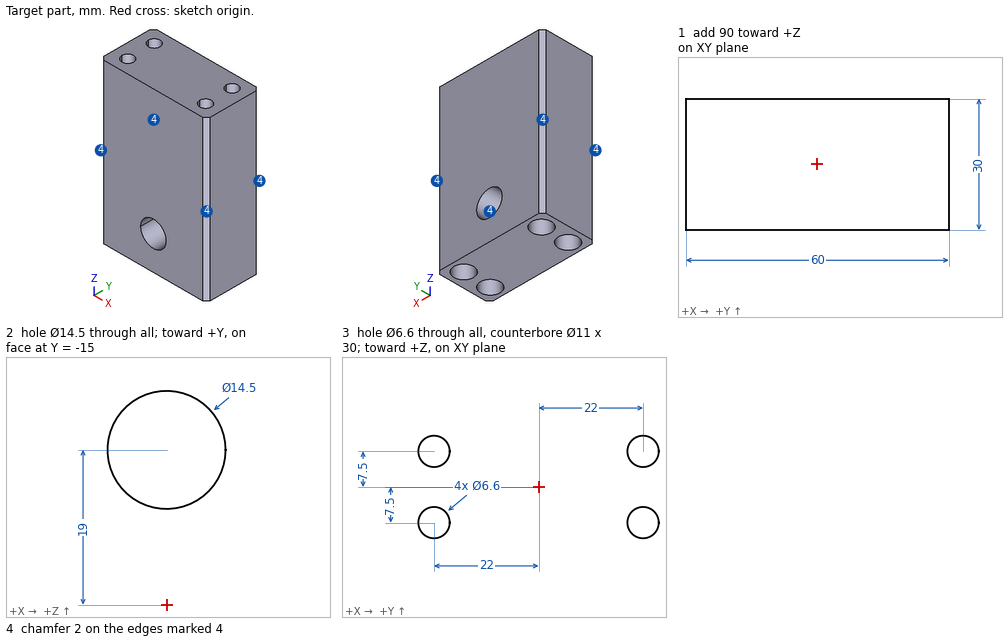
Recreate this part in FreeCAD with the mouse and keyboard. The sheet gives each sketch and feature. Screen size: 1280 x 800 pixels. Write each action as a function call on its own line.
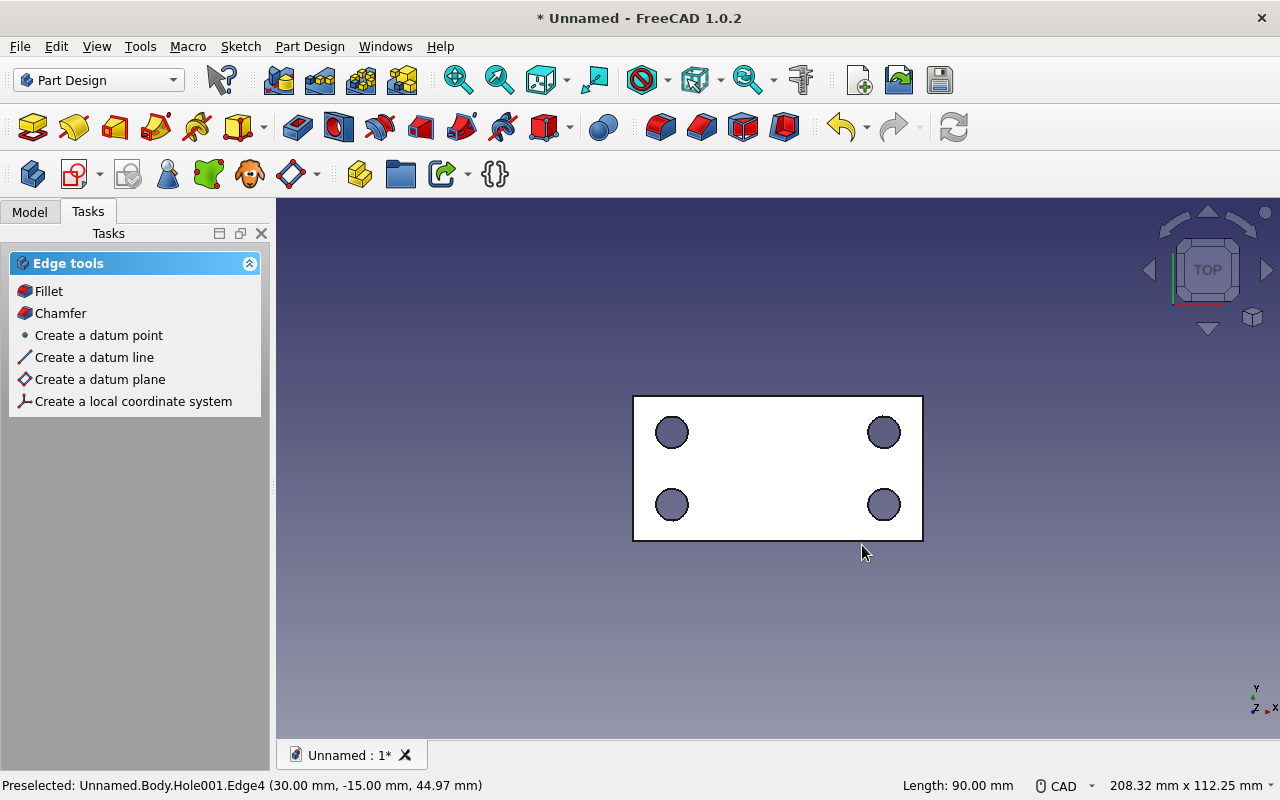
click(459, 80)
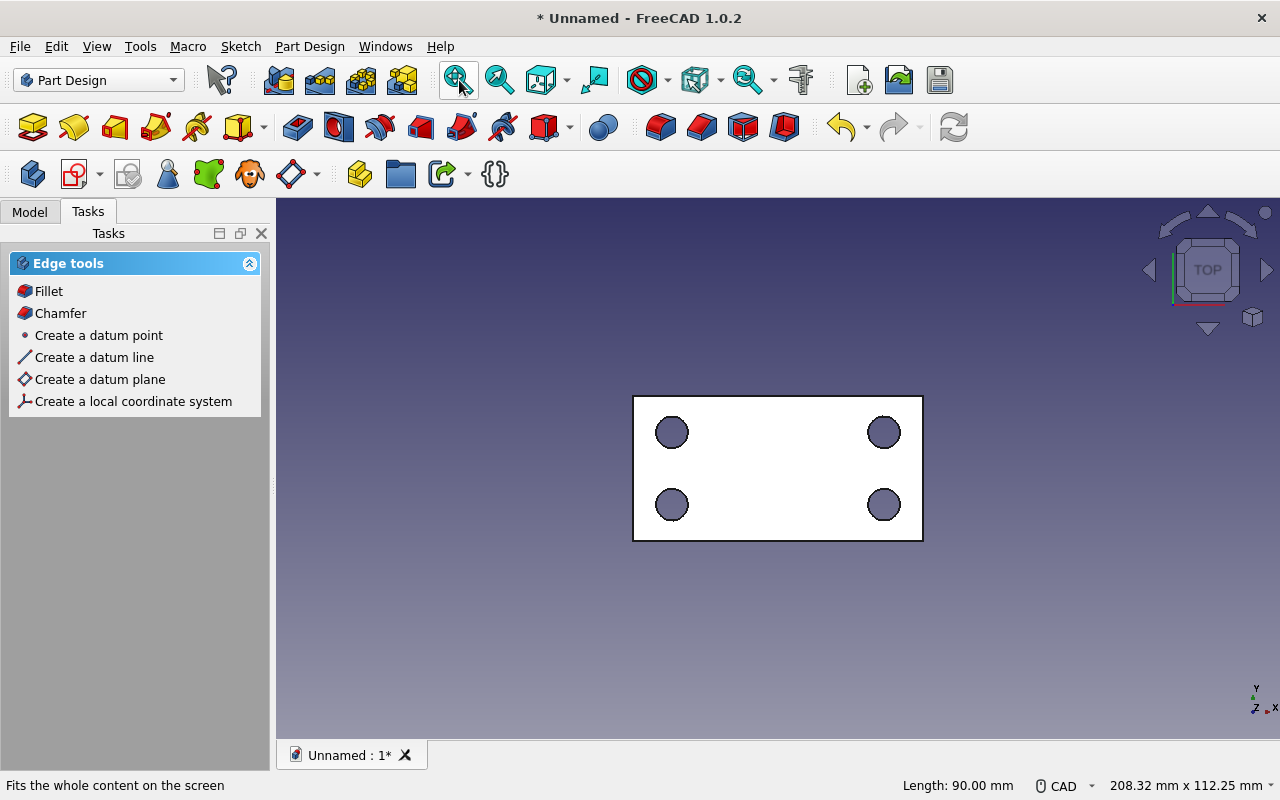
key(1)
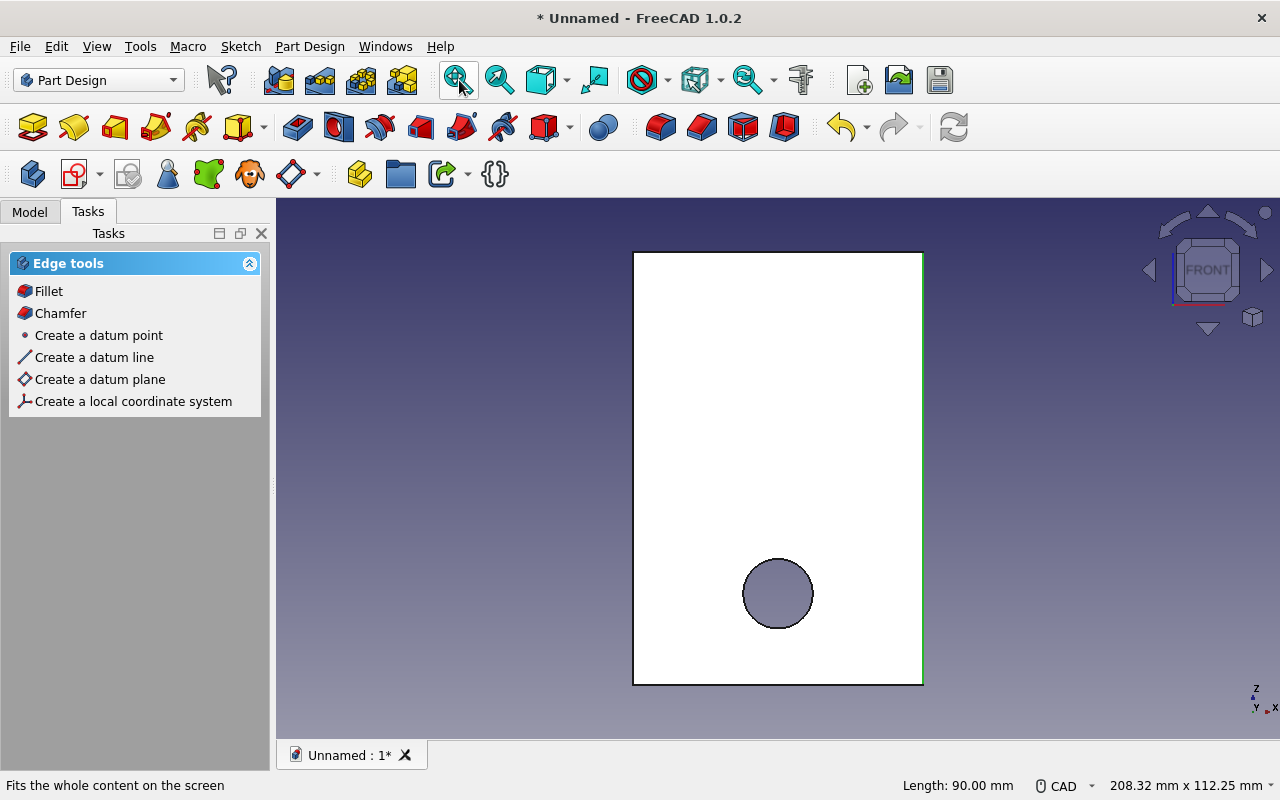
click(633, 467, ctrl)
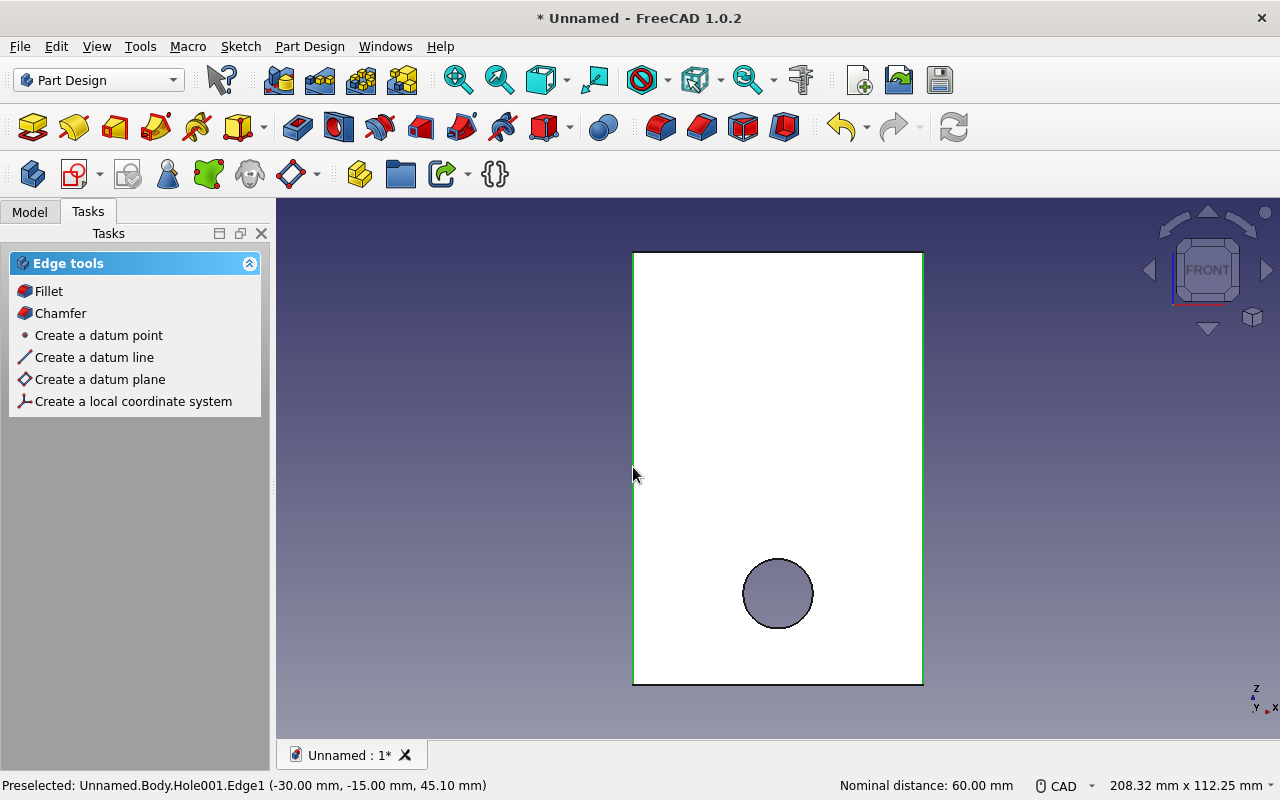
key(3)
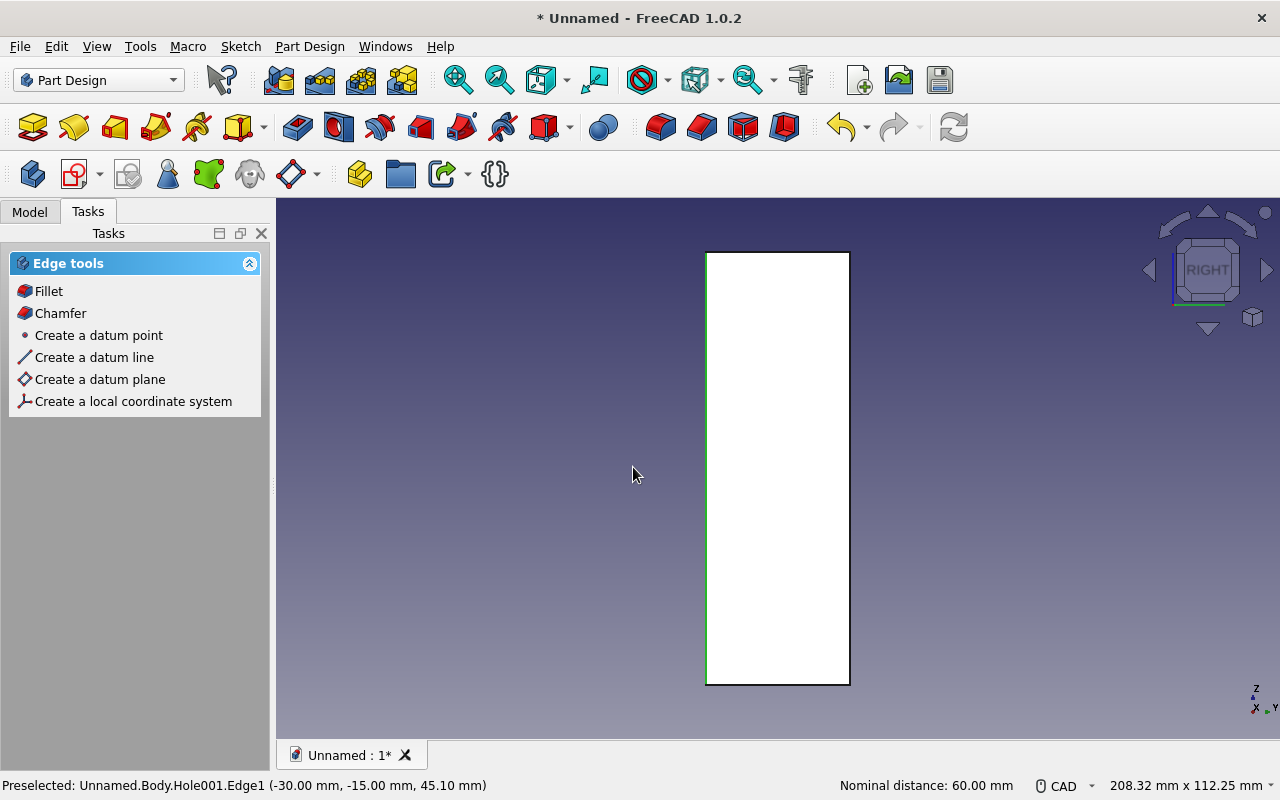
click(850, 467, ctrl)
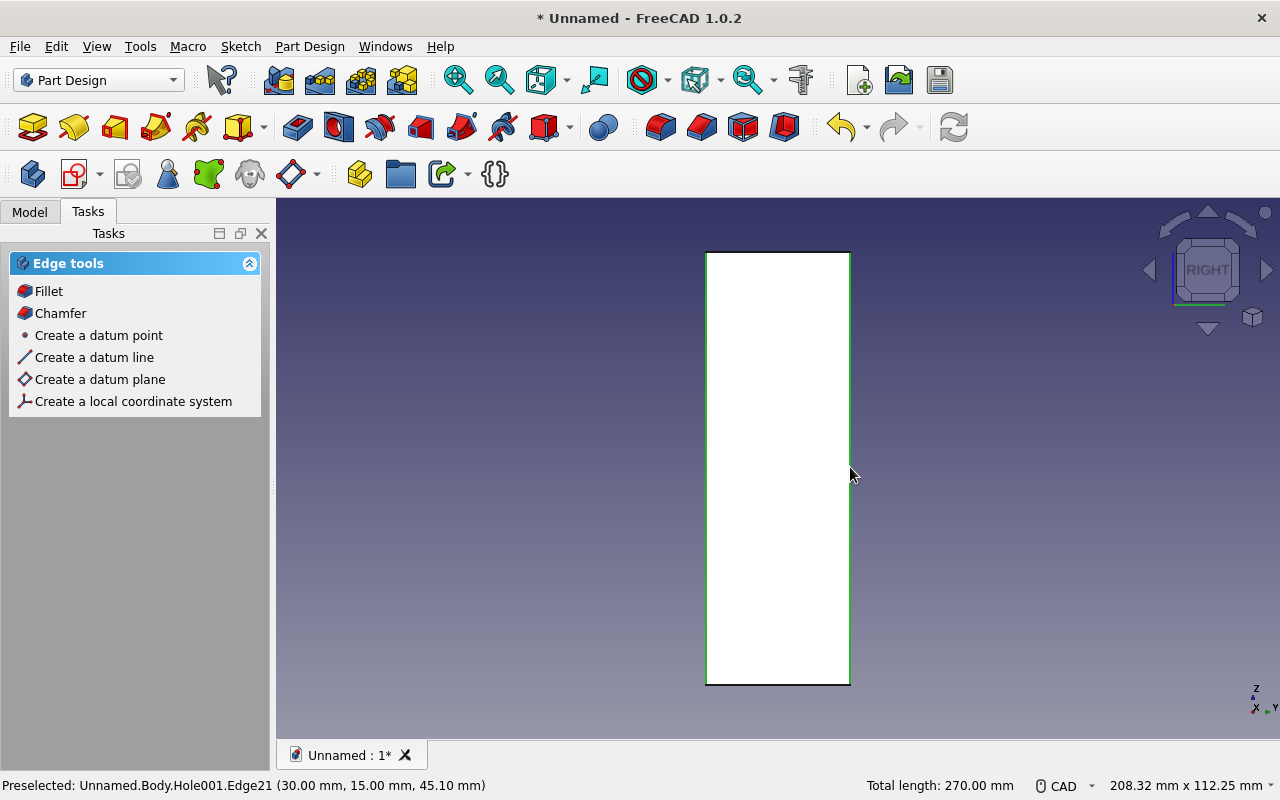
key(5)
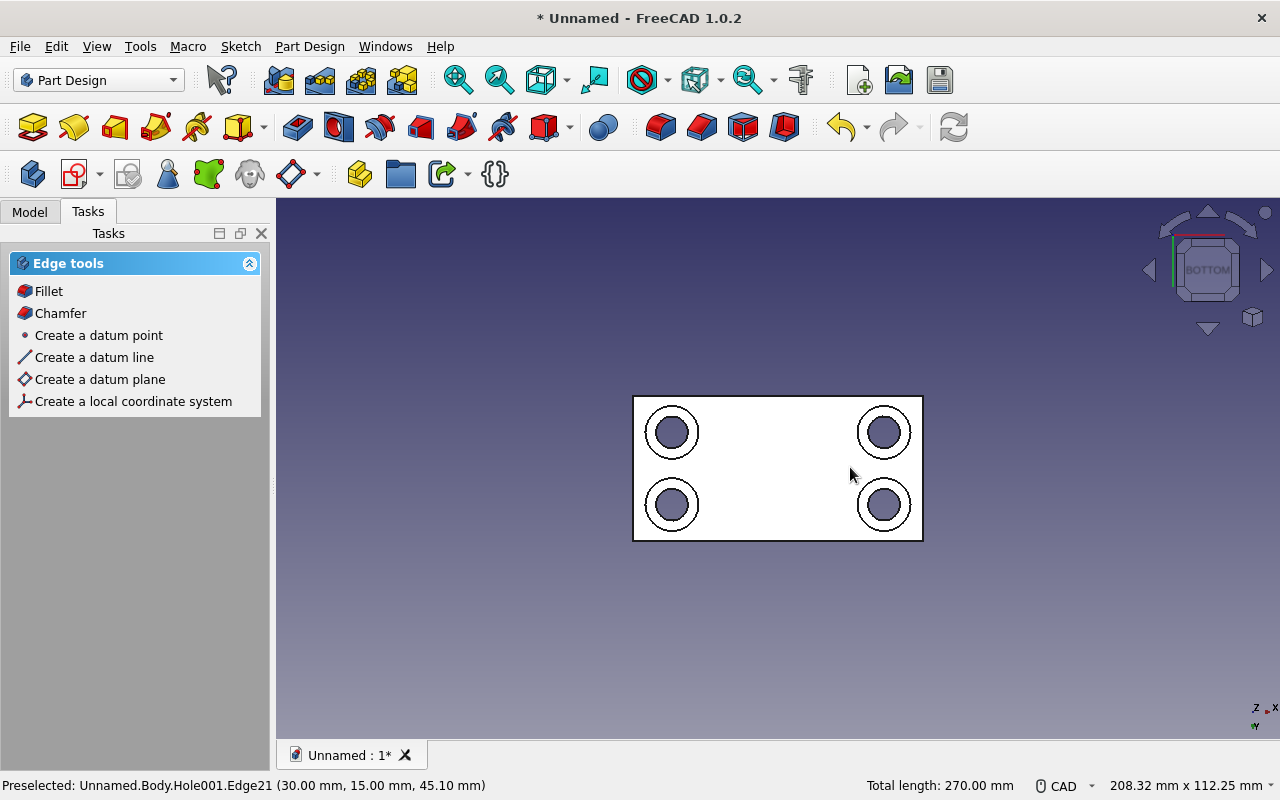
key(v)
key(f)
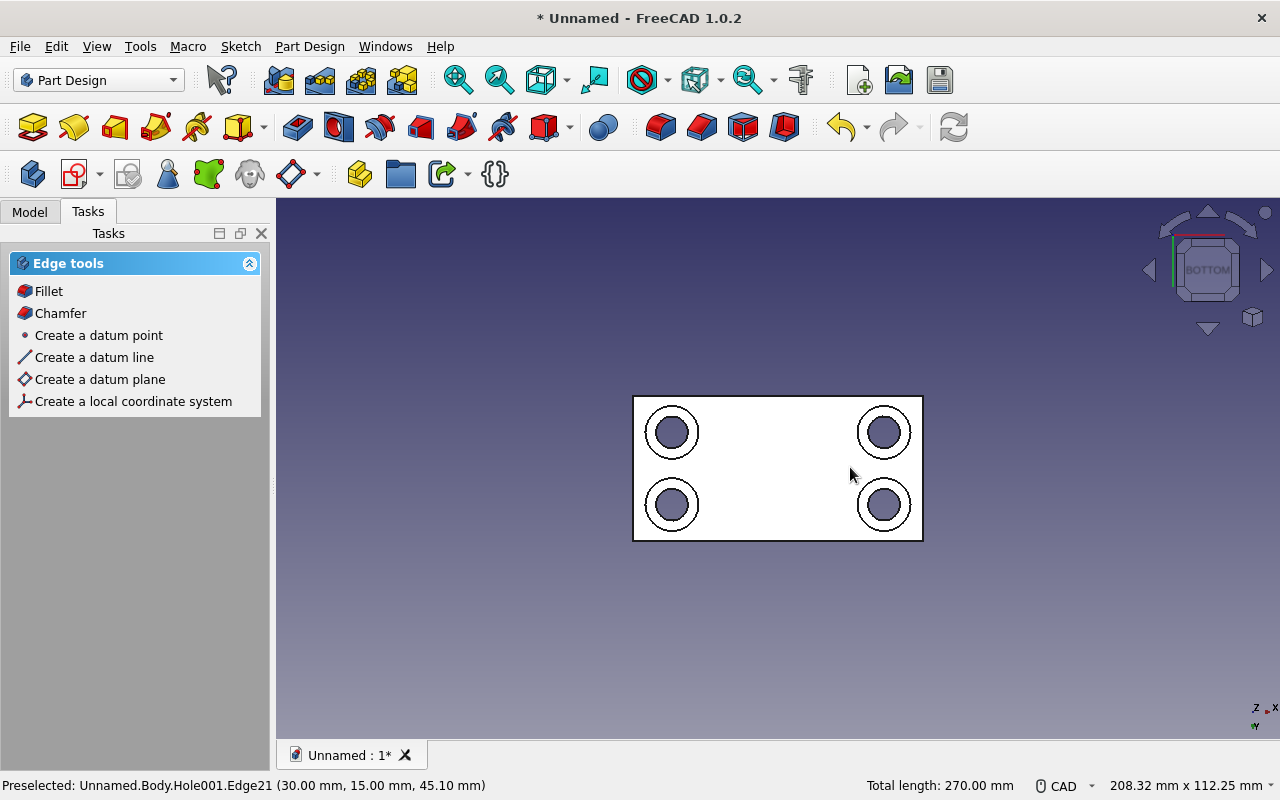
key(4)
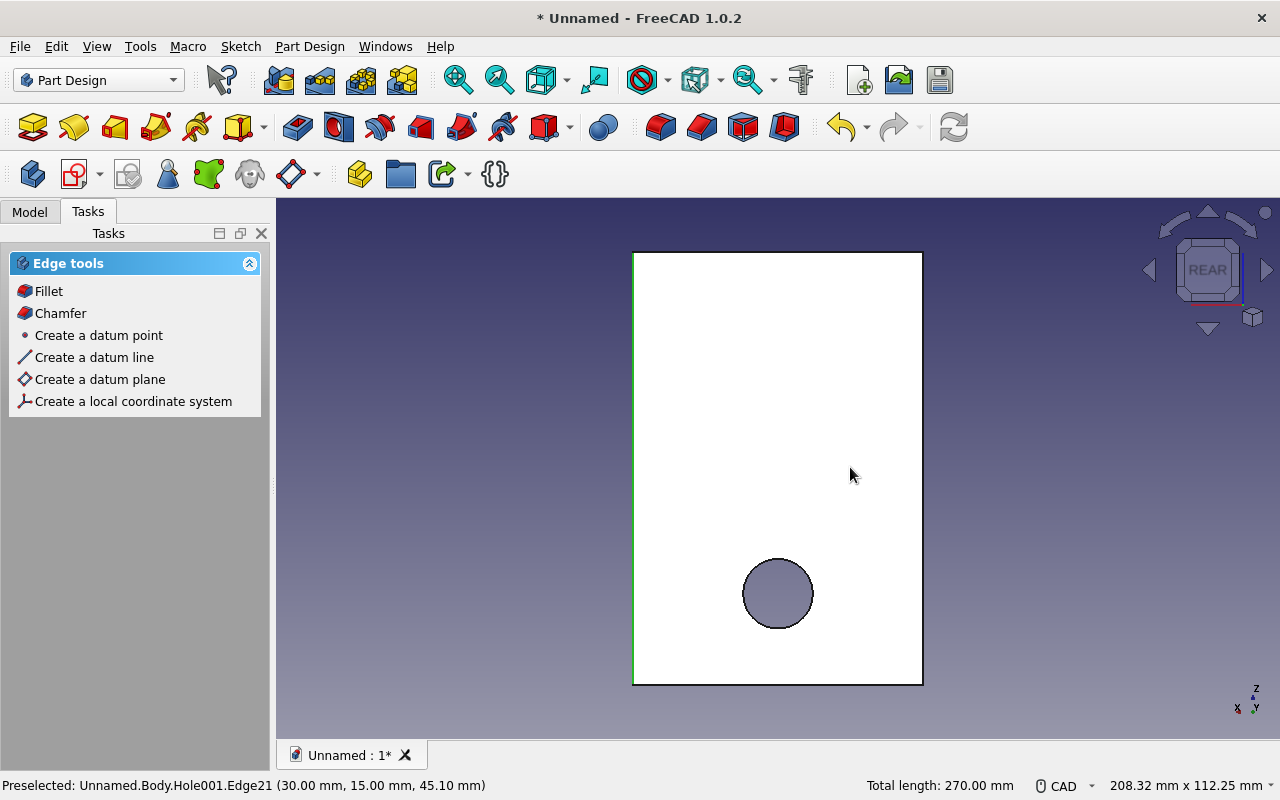
click(923, 467, ctrl)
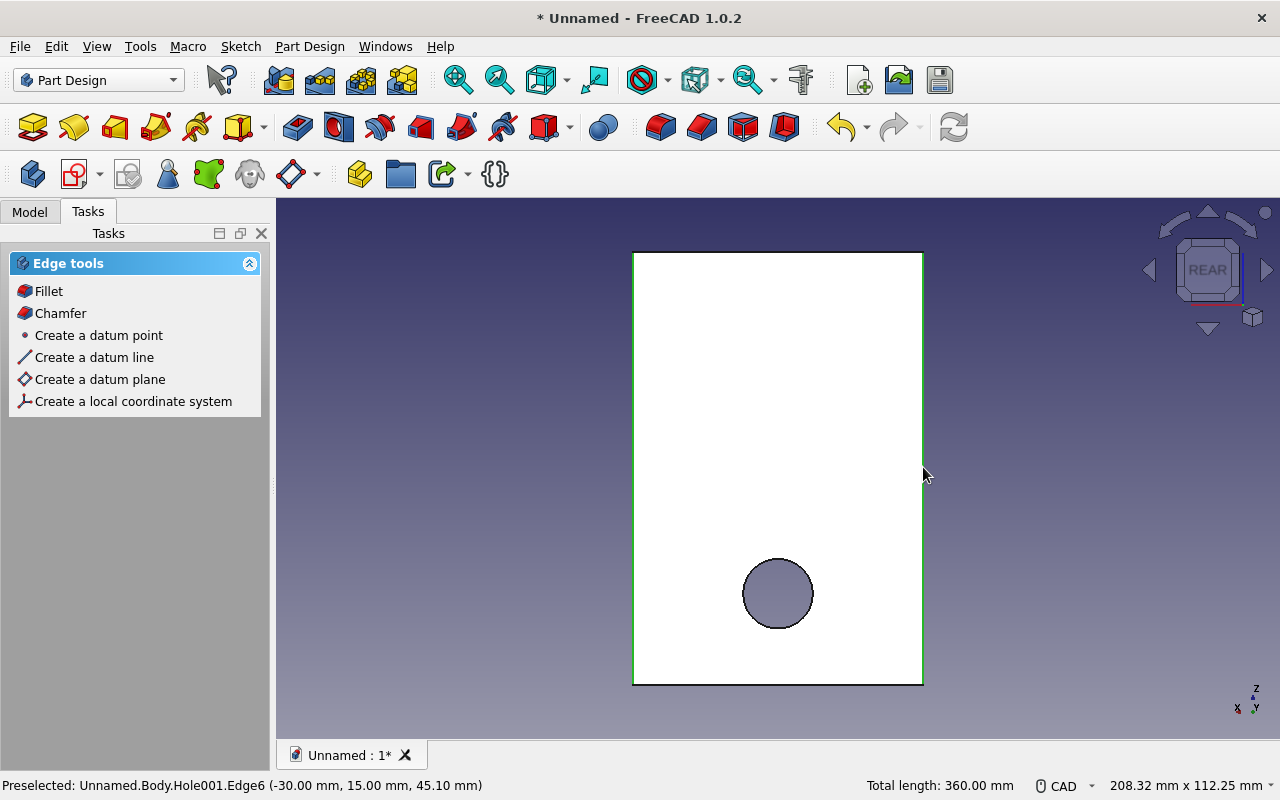
click(702, 128)